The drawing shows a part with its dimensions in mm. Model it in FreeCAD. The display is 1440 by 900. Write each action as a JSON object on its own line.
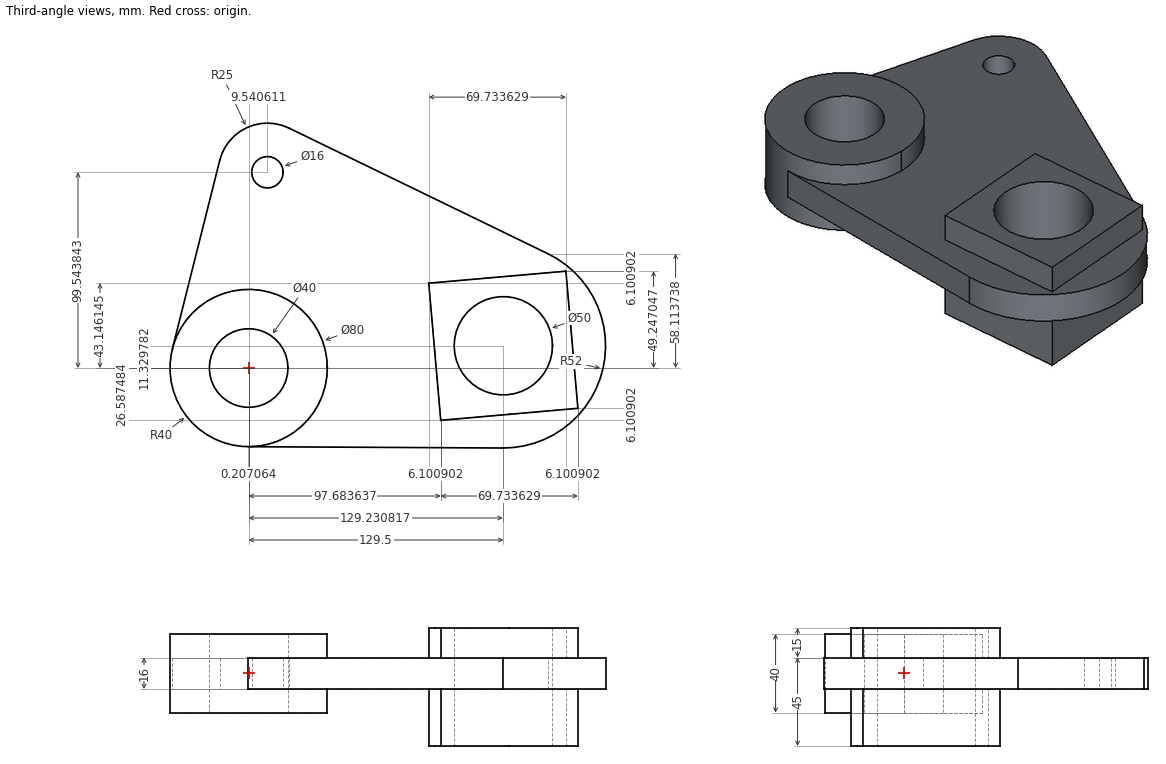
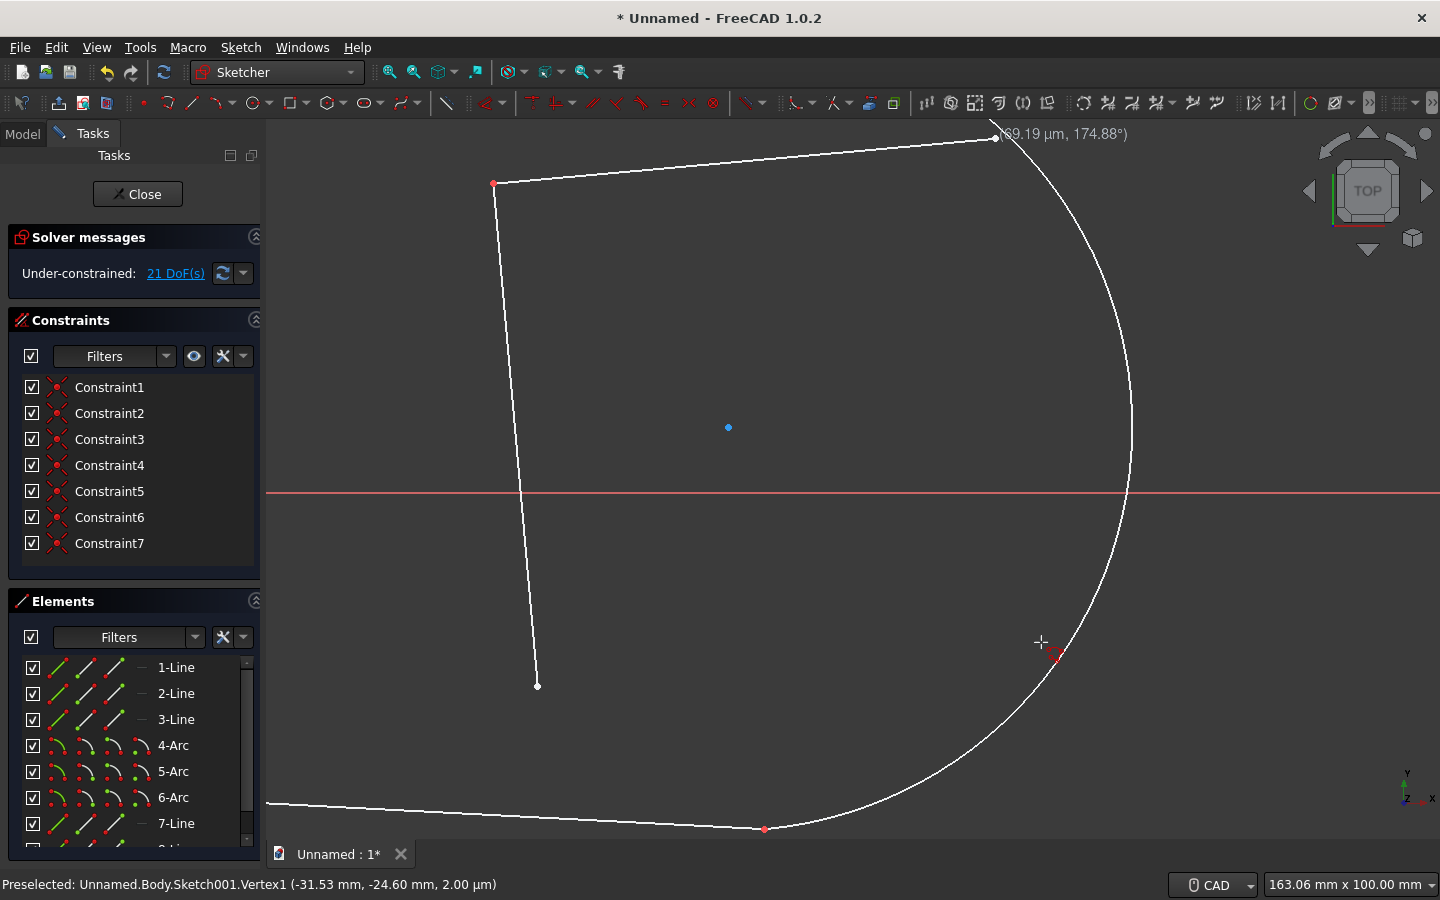
{"action": "left_click", "coordinate": [1039, 640]}
{"action": "left_click", "coordinate": [538, 687]}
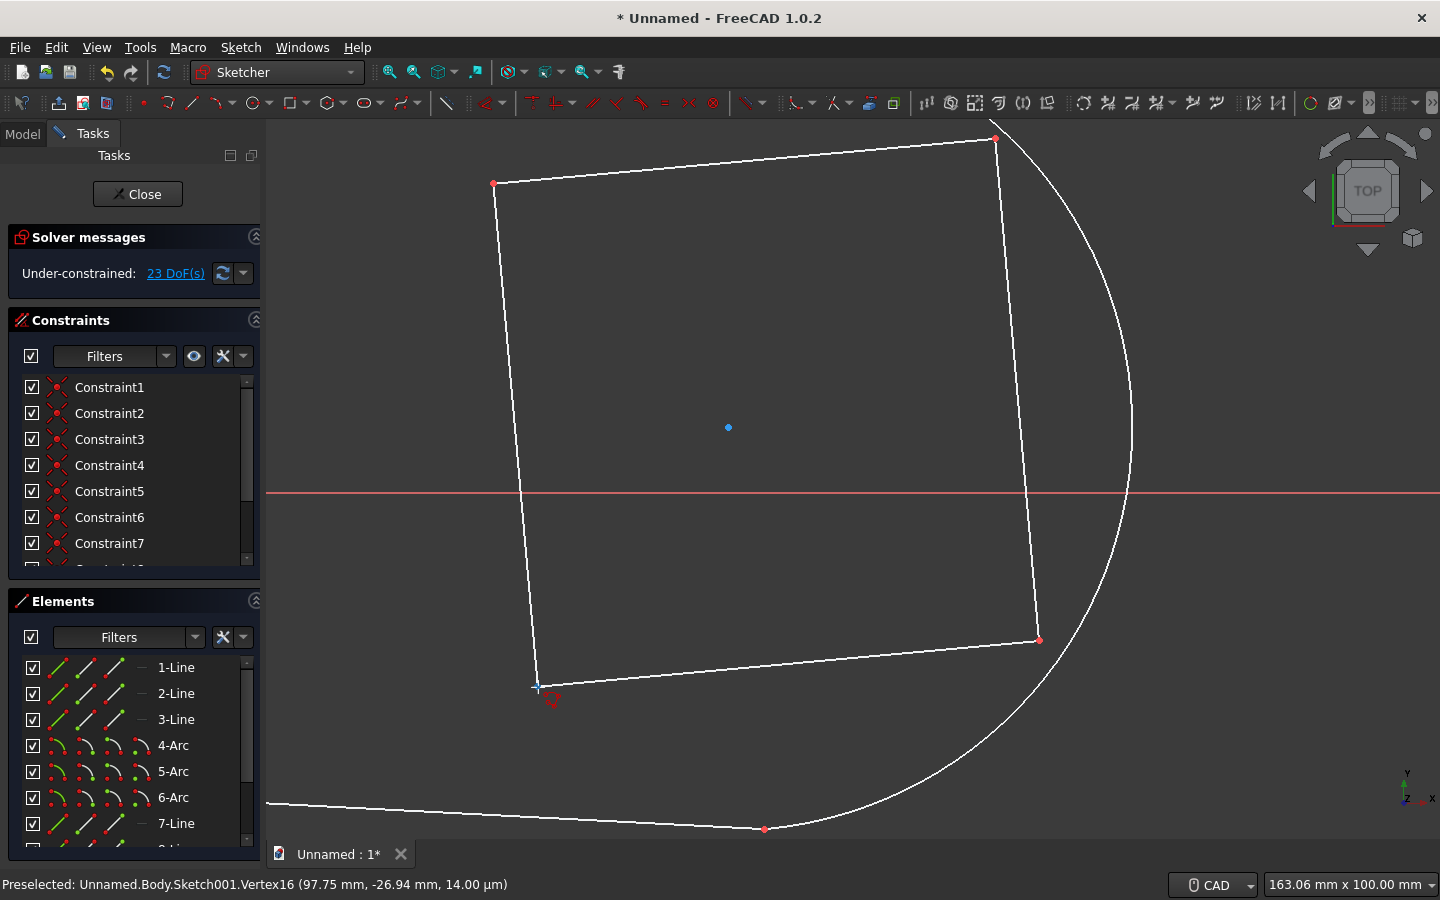
{"action": "key", "text": "g c"}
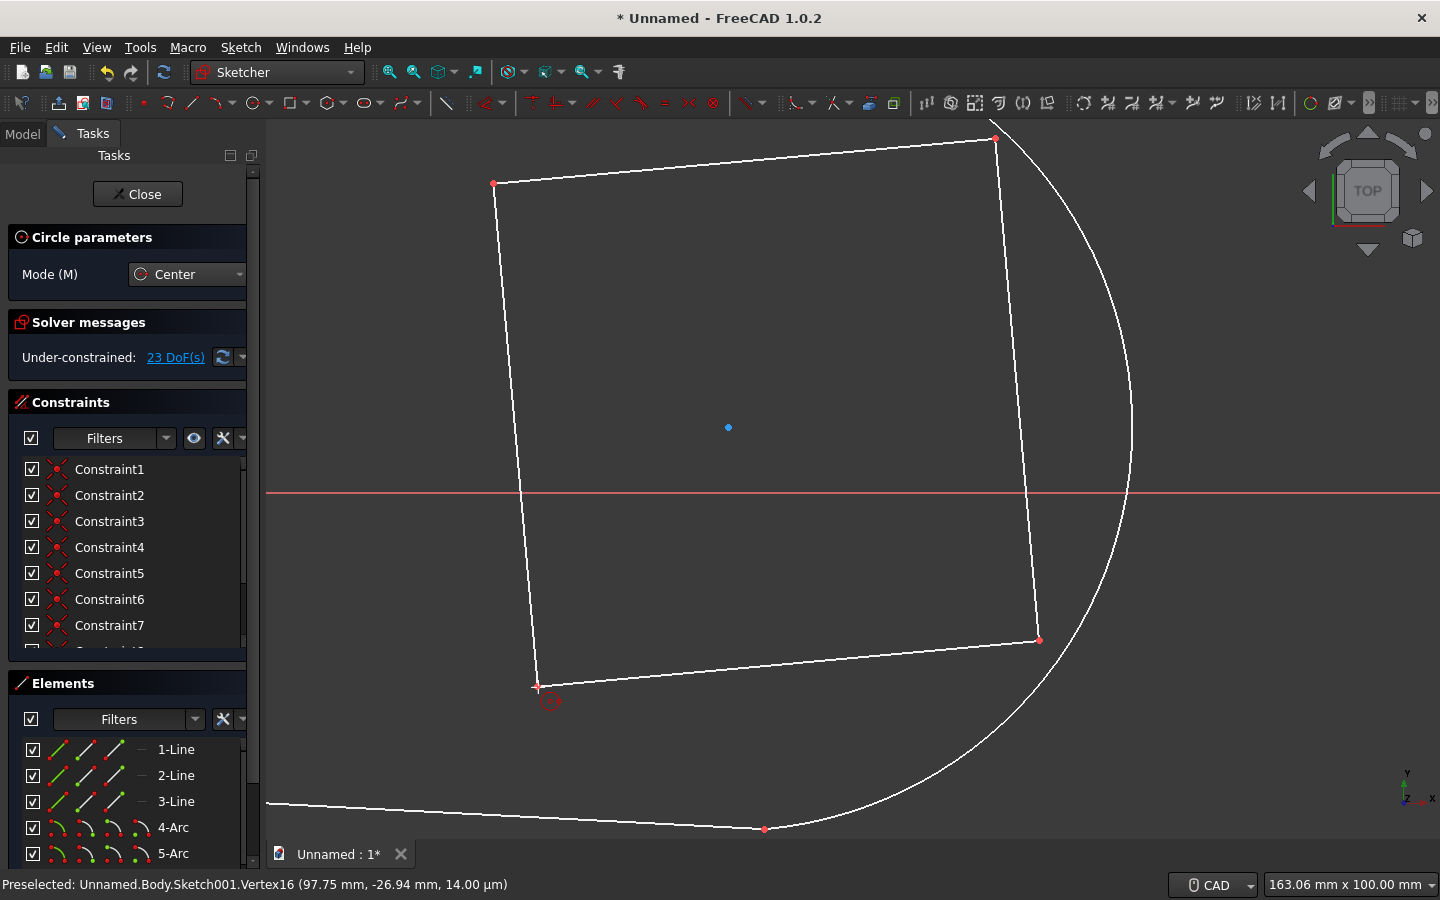
{"action": "scroll", "coordinate": [1041, 642], "scroll_direction": "down", "scroll_amount": 5}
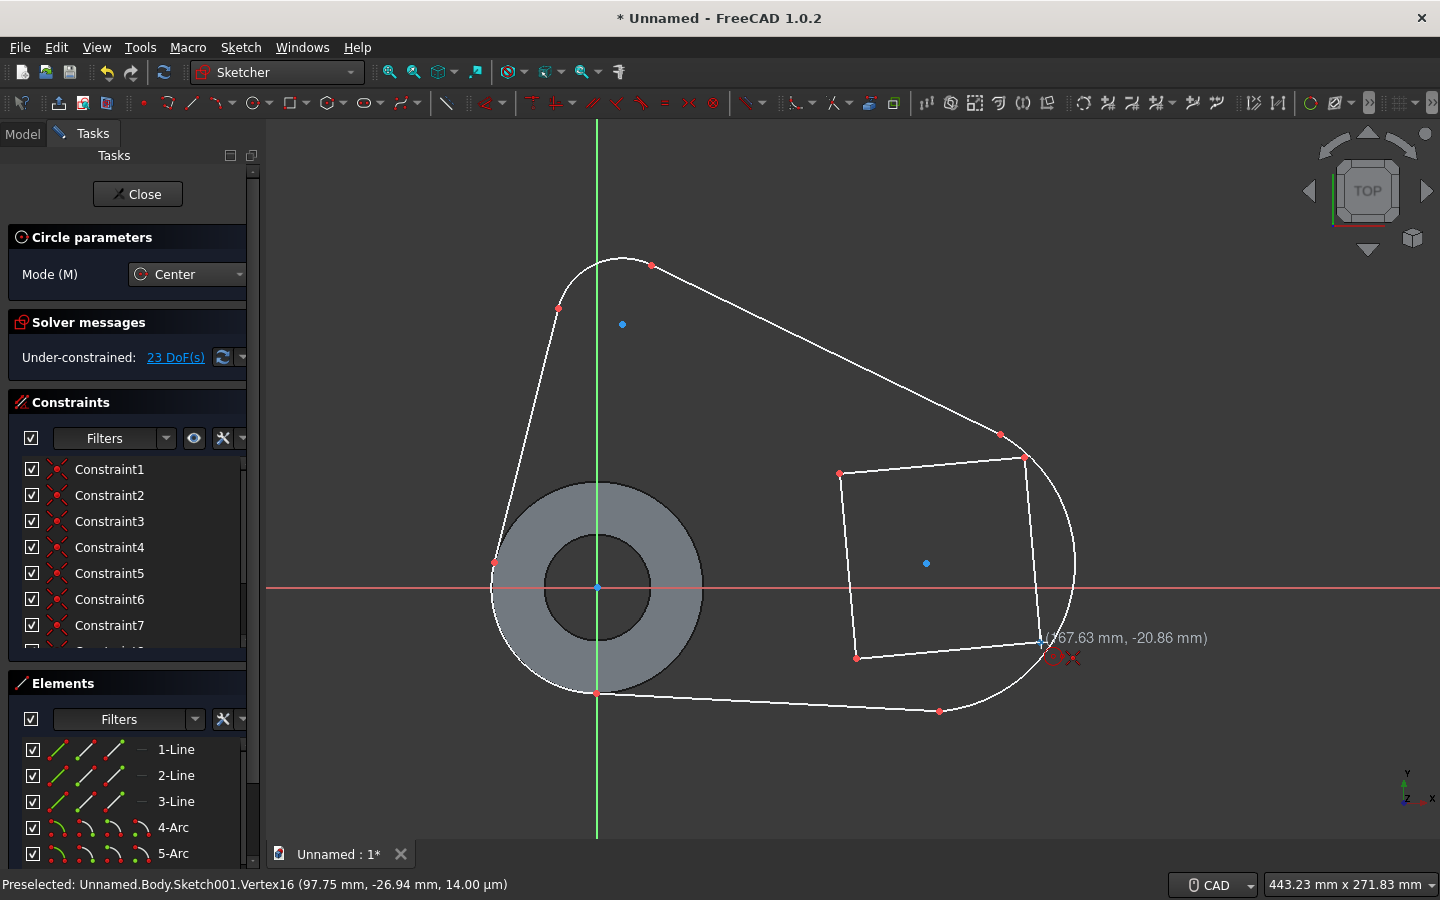
{"action": "left_click", "coordinate": [597, 588]}
{"action": "left_click", "coordinate": [635, 550]}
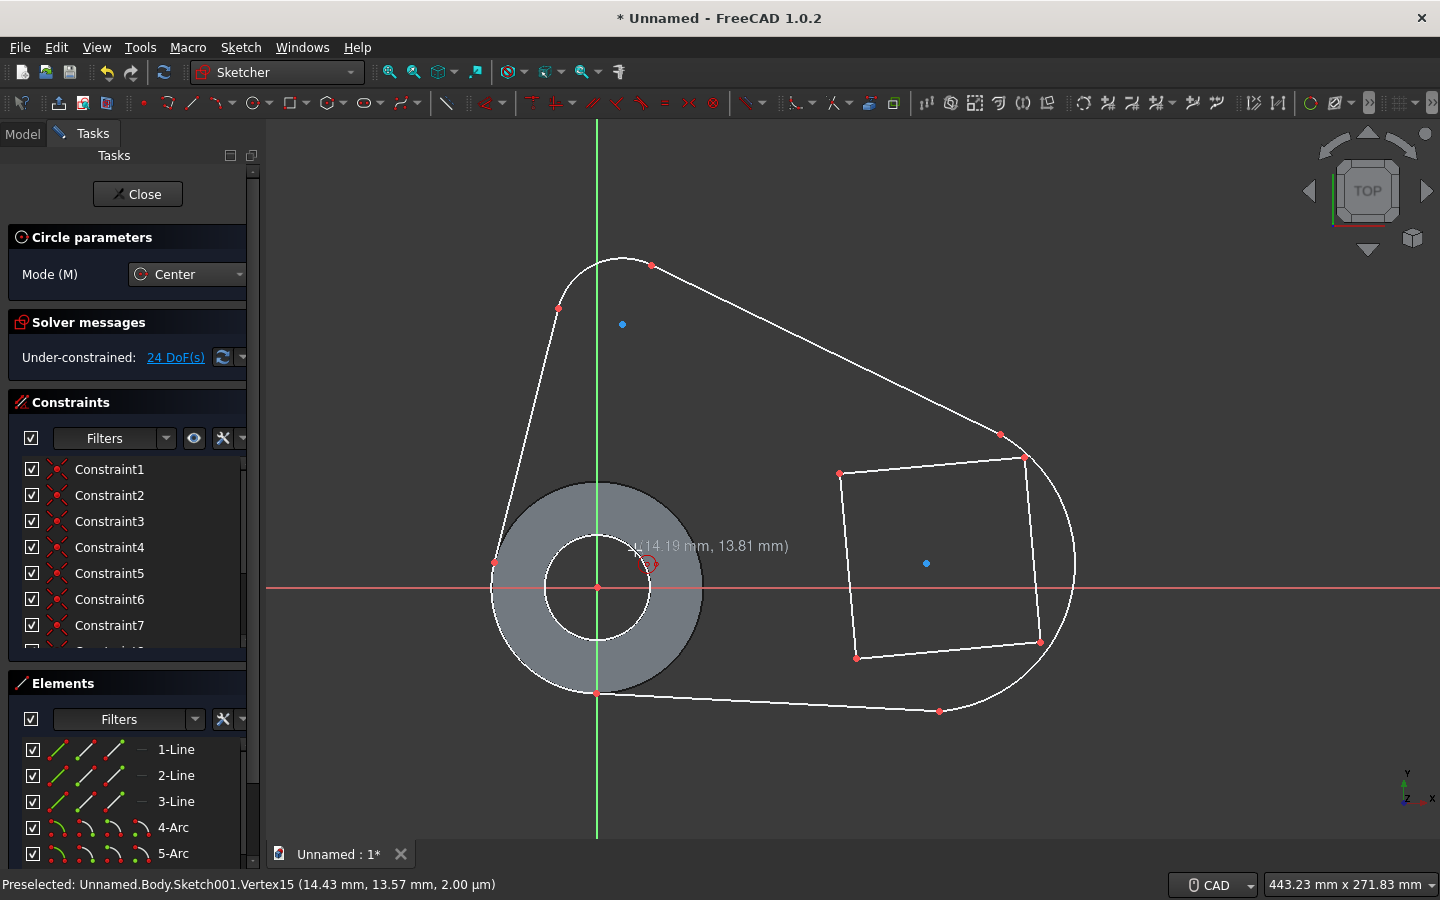
{"action": "left_click", "coordinate": [623, 324]}
{"action": "left_click", "coordinate": [638, 309]}
{"action": "key", "text": "Escape"}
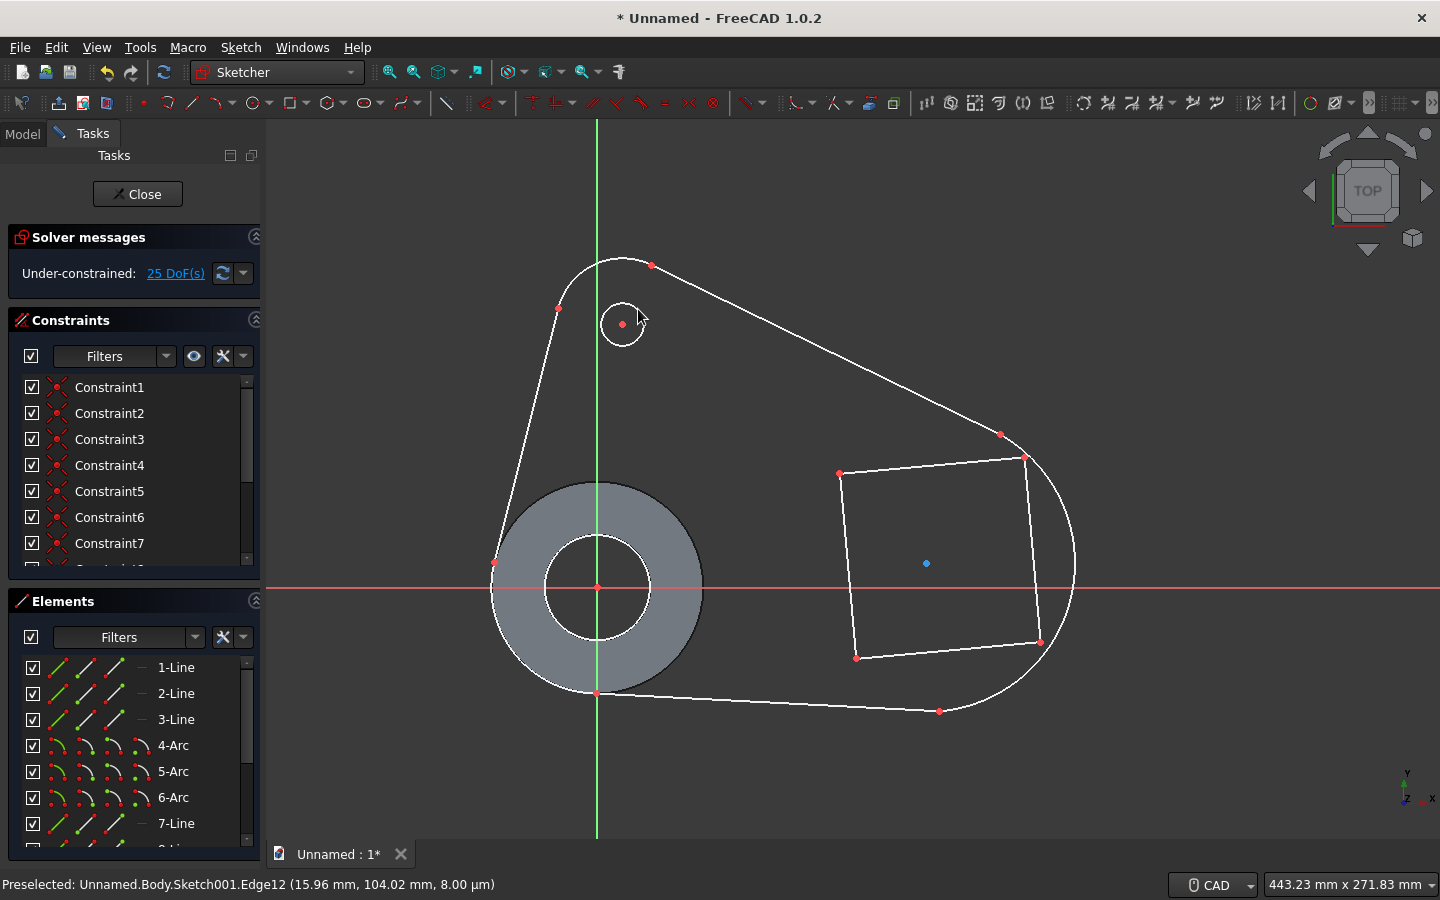
{"action": "left_click", "coordinate": [700, 699]}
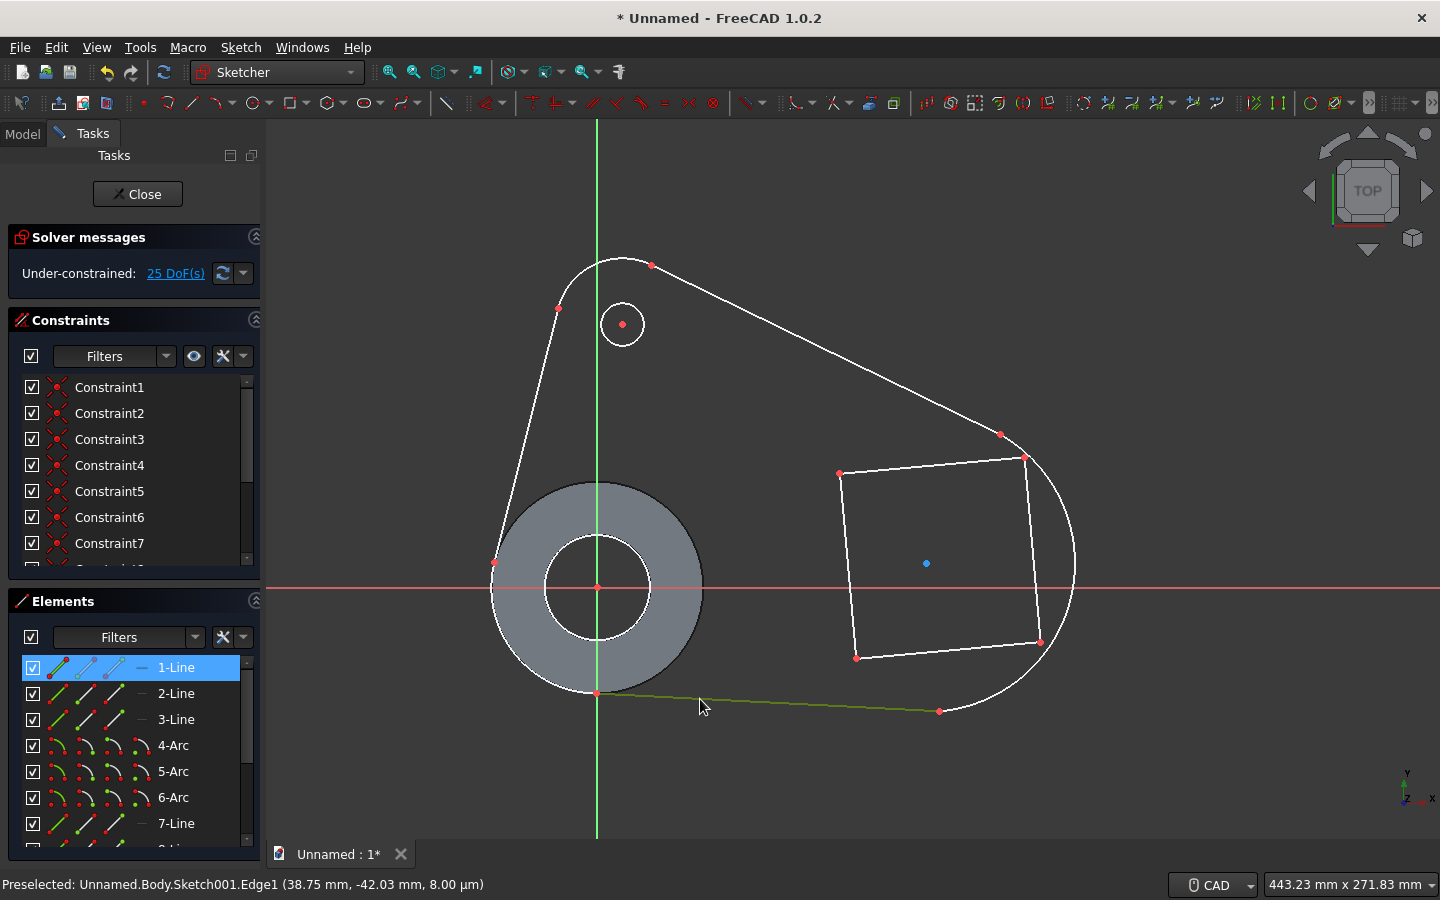
{"action": "left_click", "coordinate": [496, 619]}